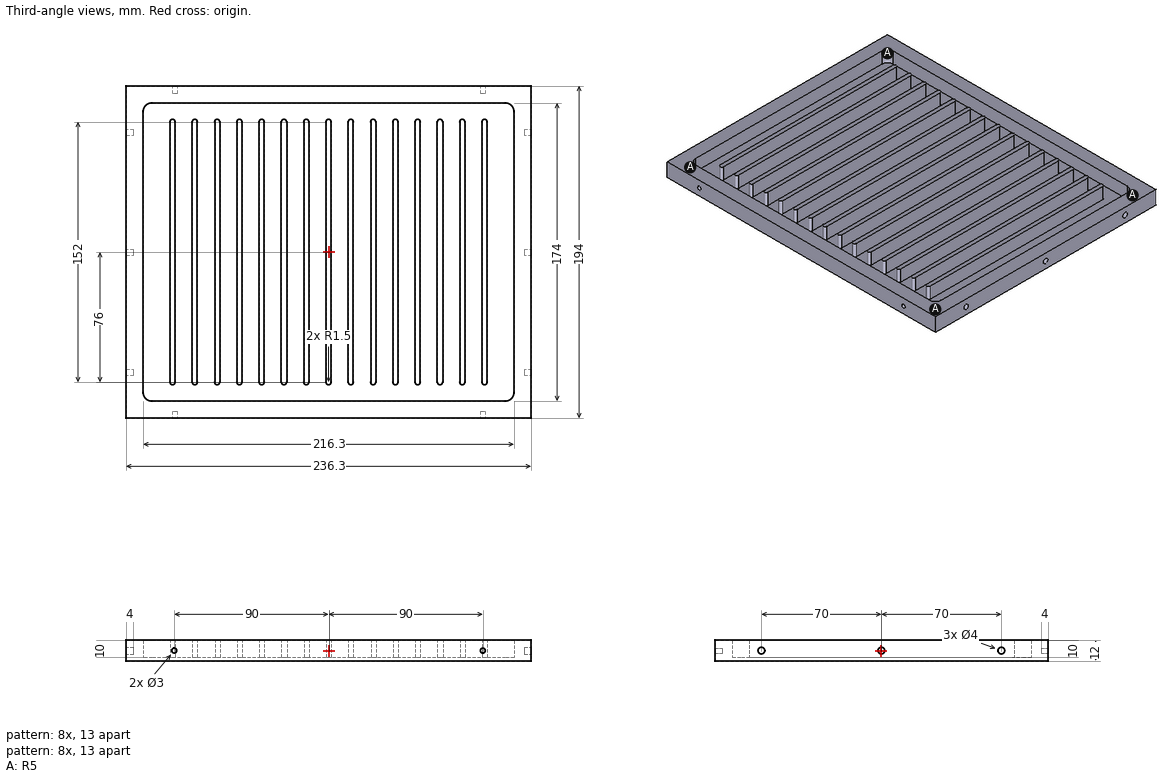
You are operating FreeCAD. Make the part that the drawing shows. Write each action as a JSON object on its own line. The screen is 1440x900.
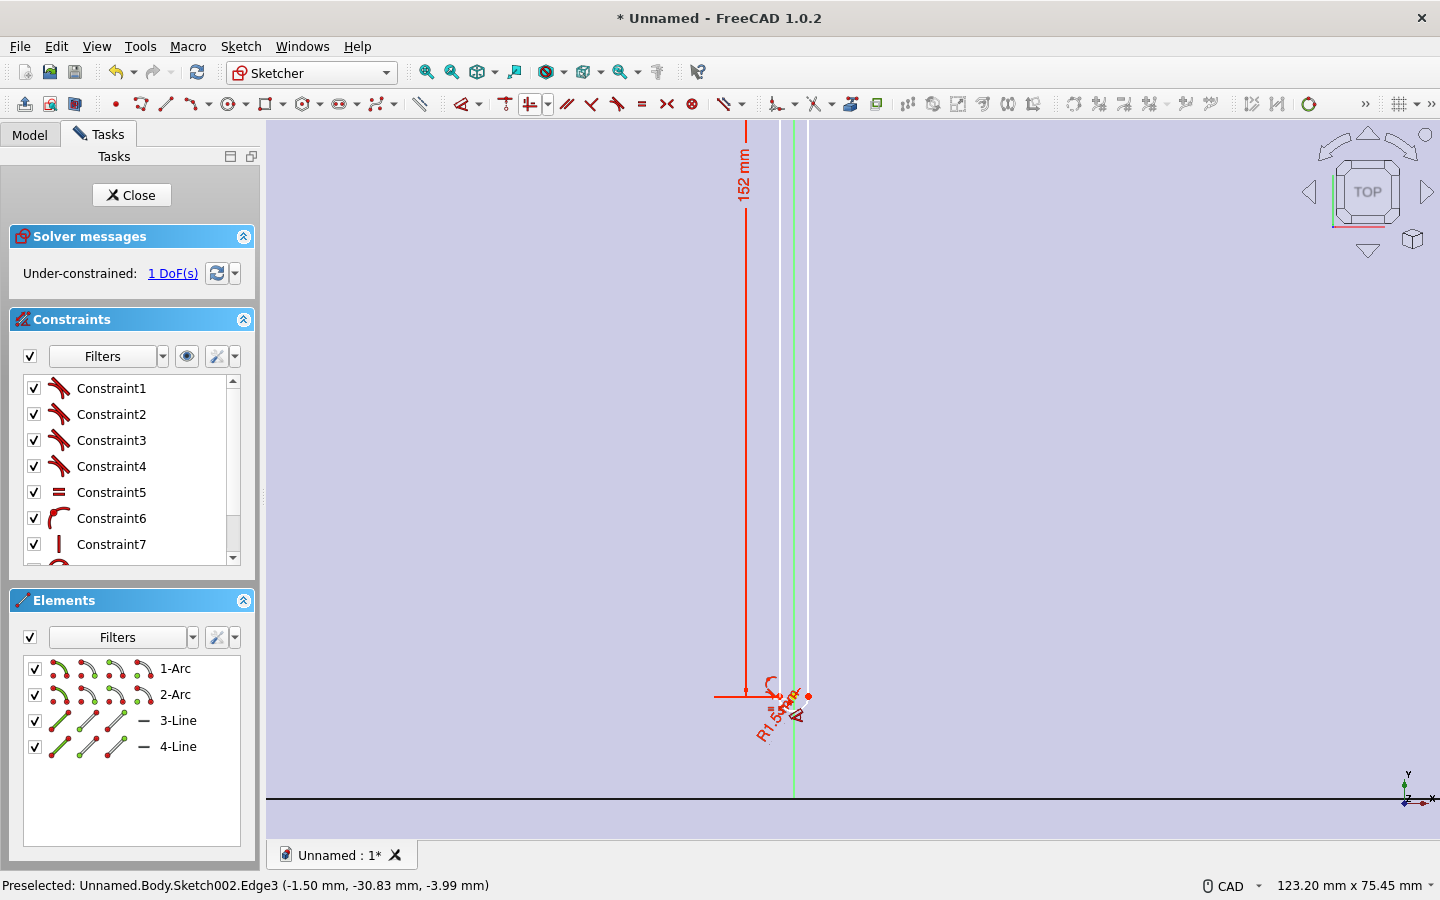
{"action": "left_click", "coordinate": [780, 697]}
{"action": "left_click", "coordinate": [746, 422]}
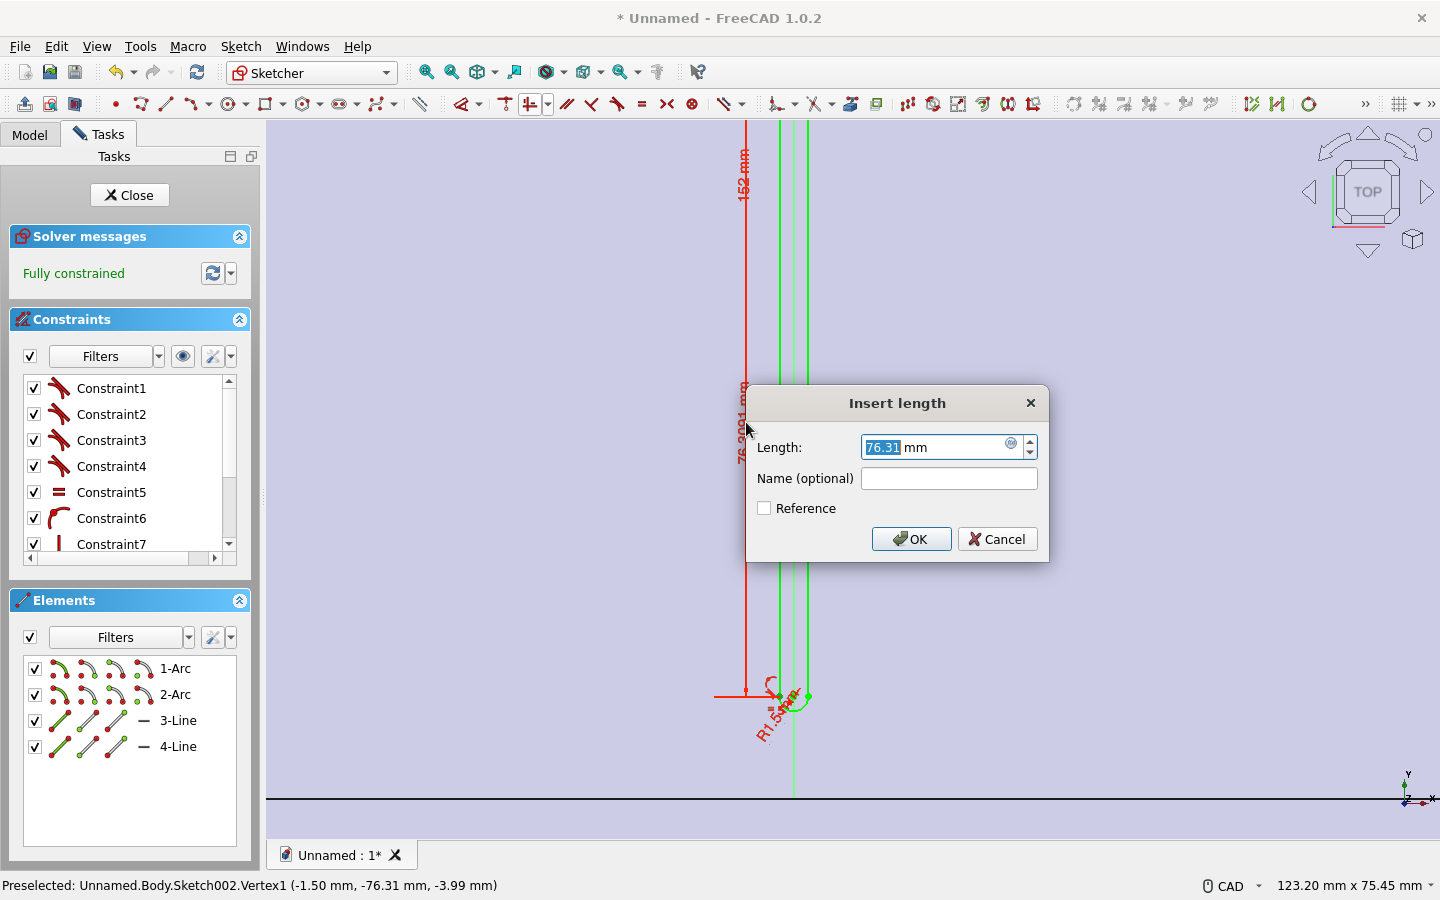
{"action": "type", "text": "76"}
{"action": "key", "text": "Return"}
{"action": "key", "text": "Escape"}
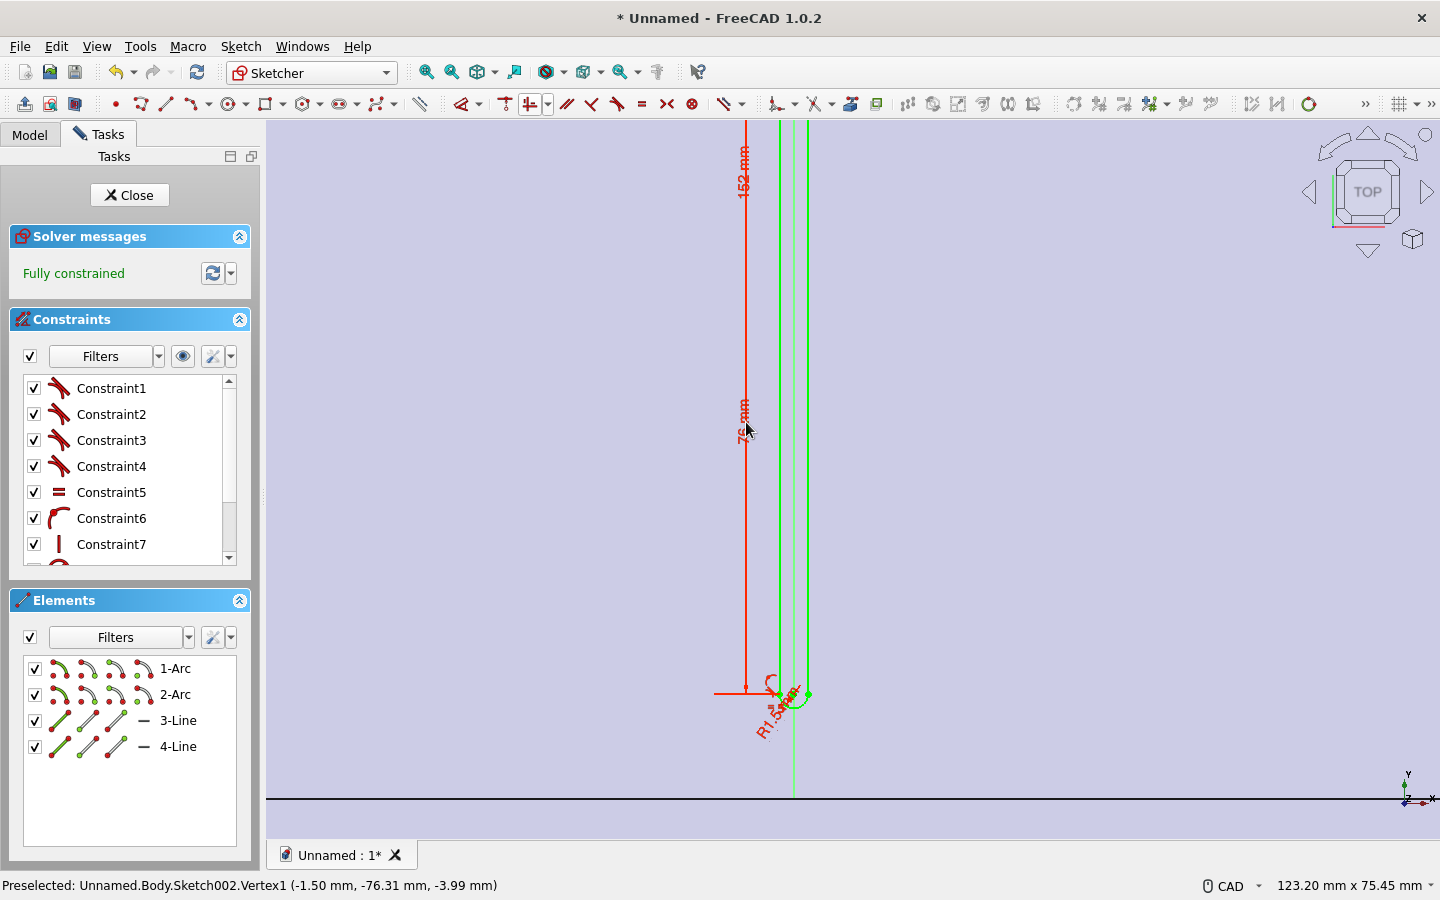
{"action": "left_click", "coordinate": [130, 195]}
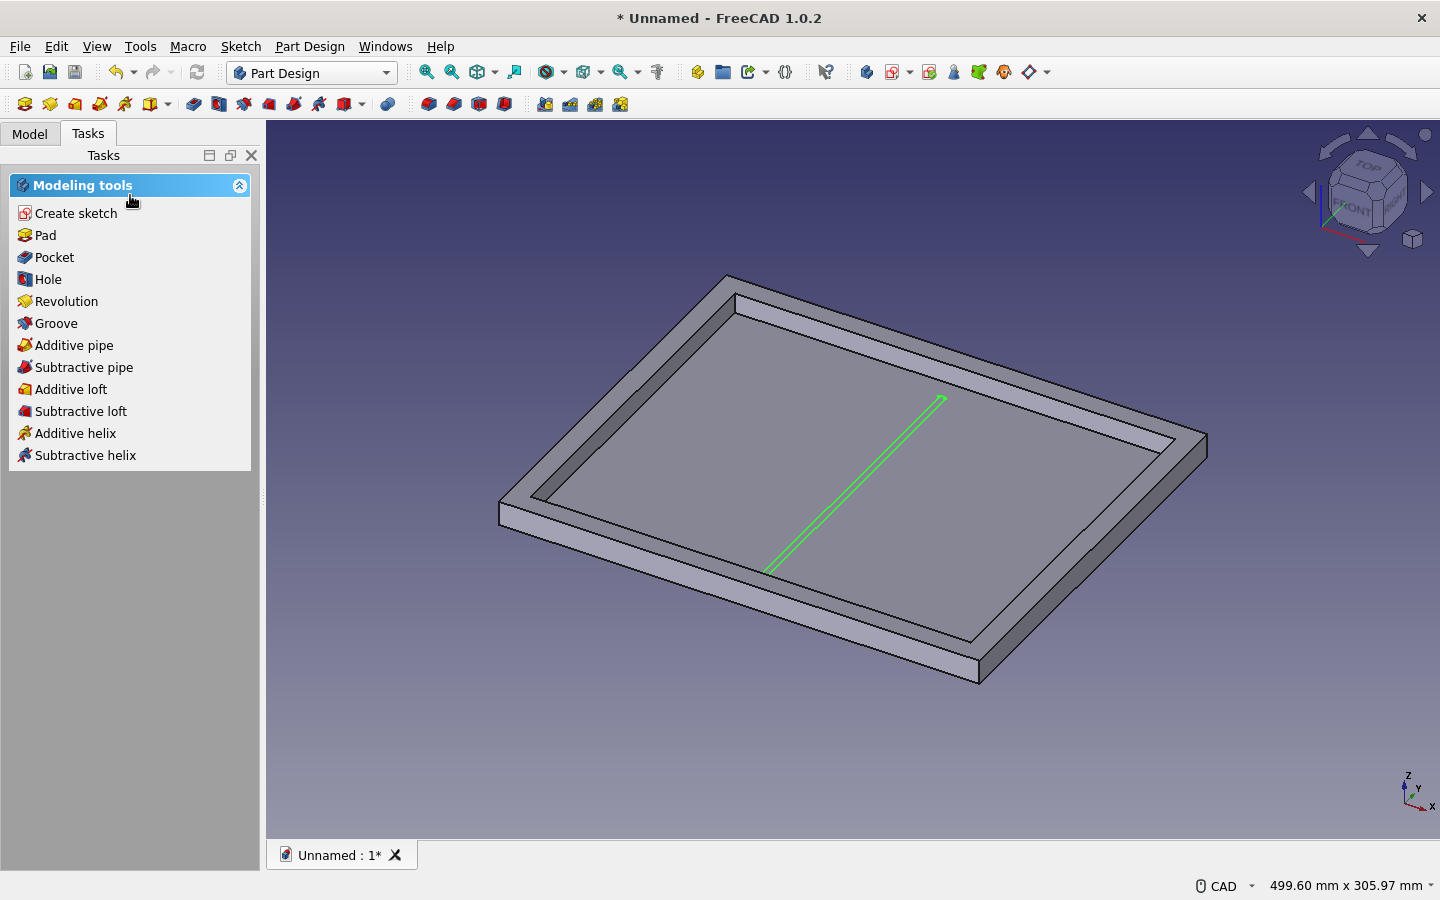
{"action": "left_click", "coordinate": [25, 104]}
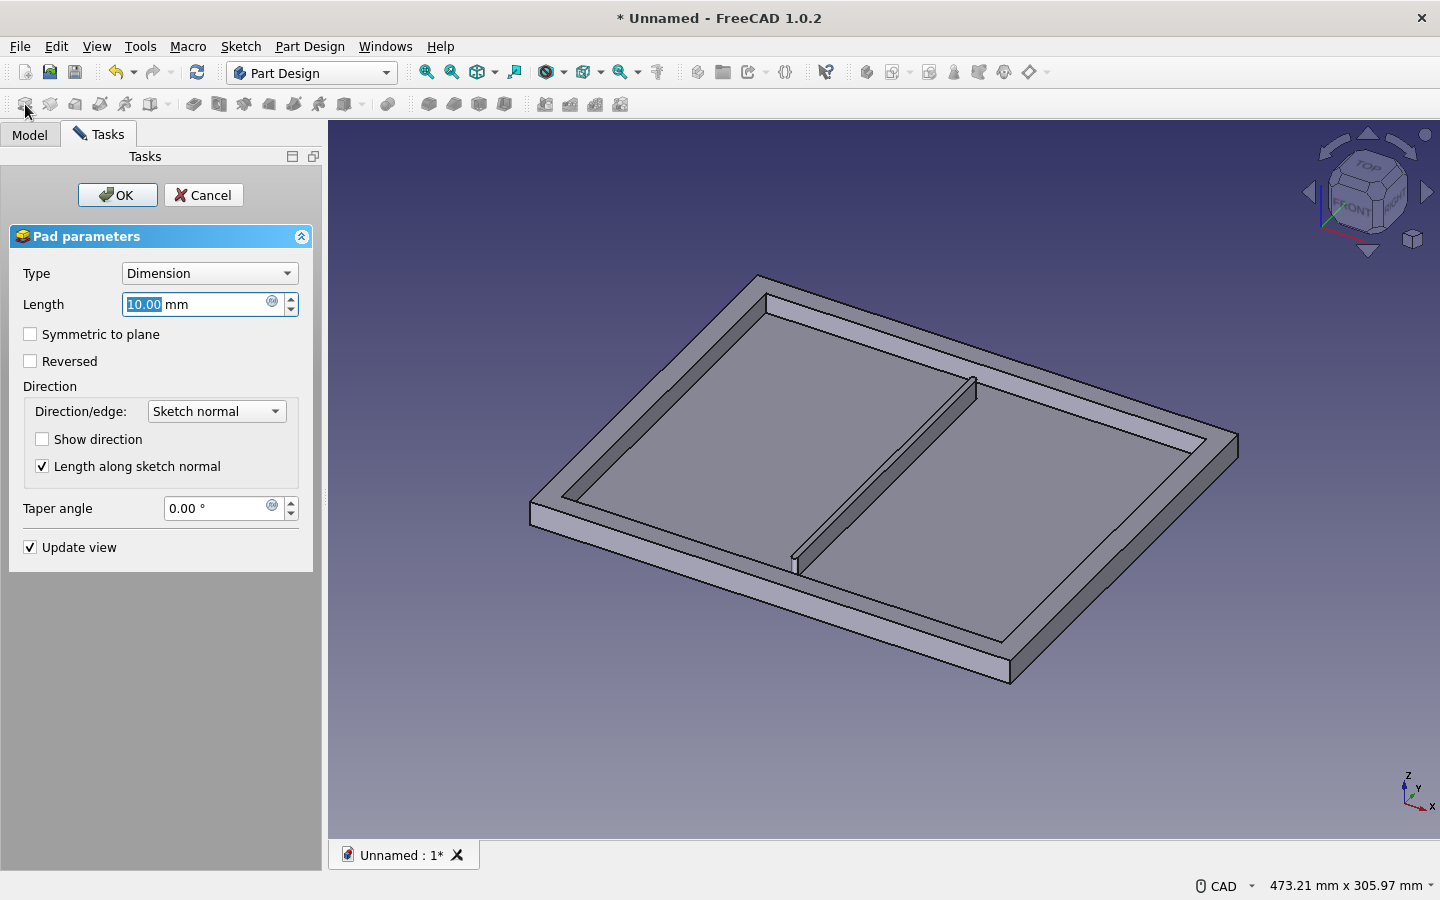
{"action": "type", "text": "10"}
{"action": "key", "text": "Tab"}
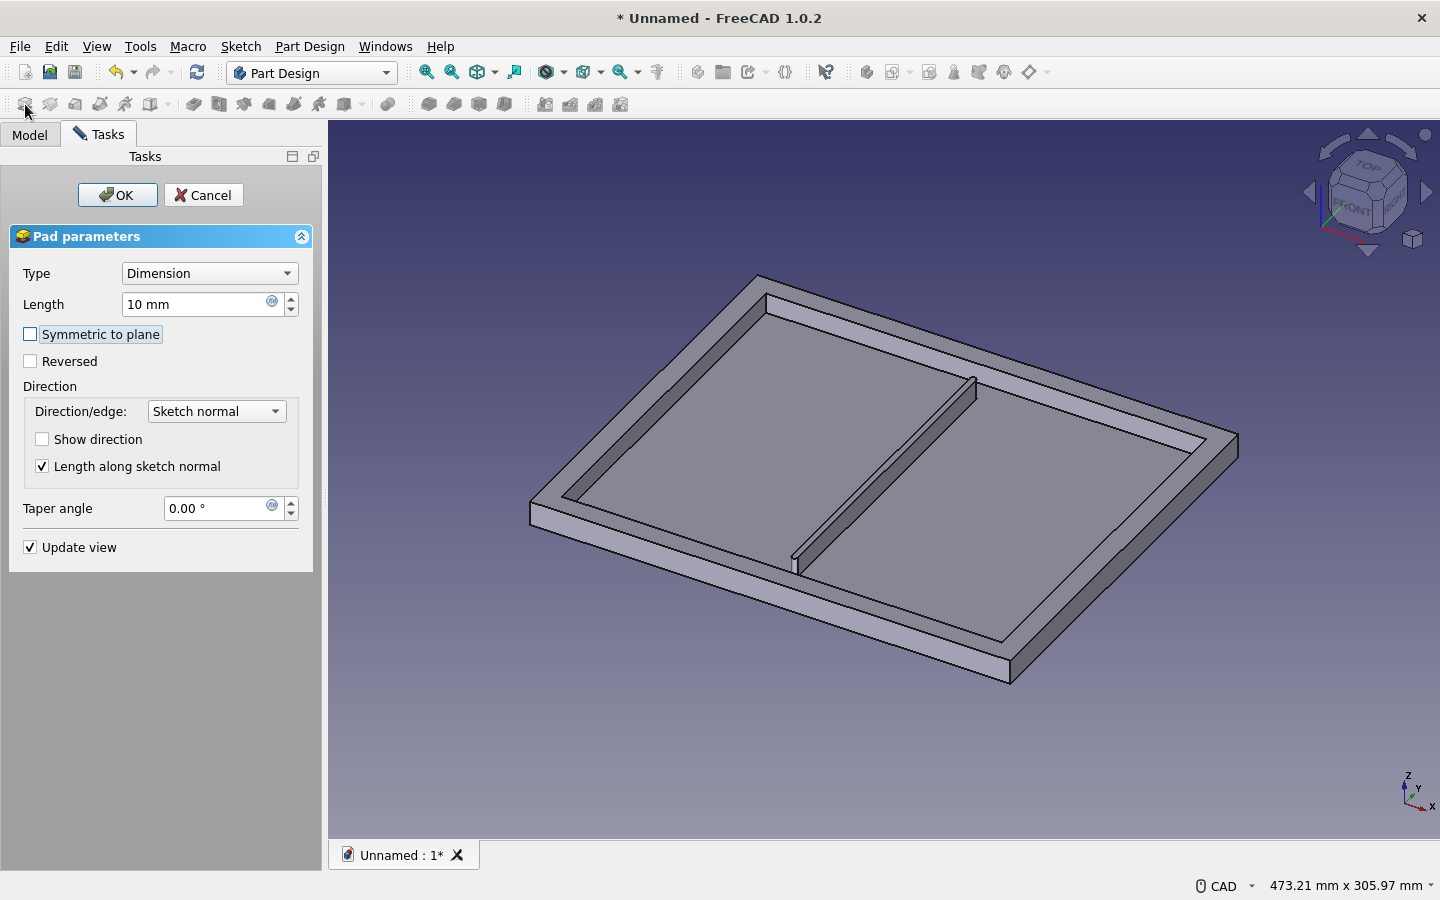
{"action": "left_click", "coordinate": [118, 195]}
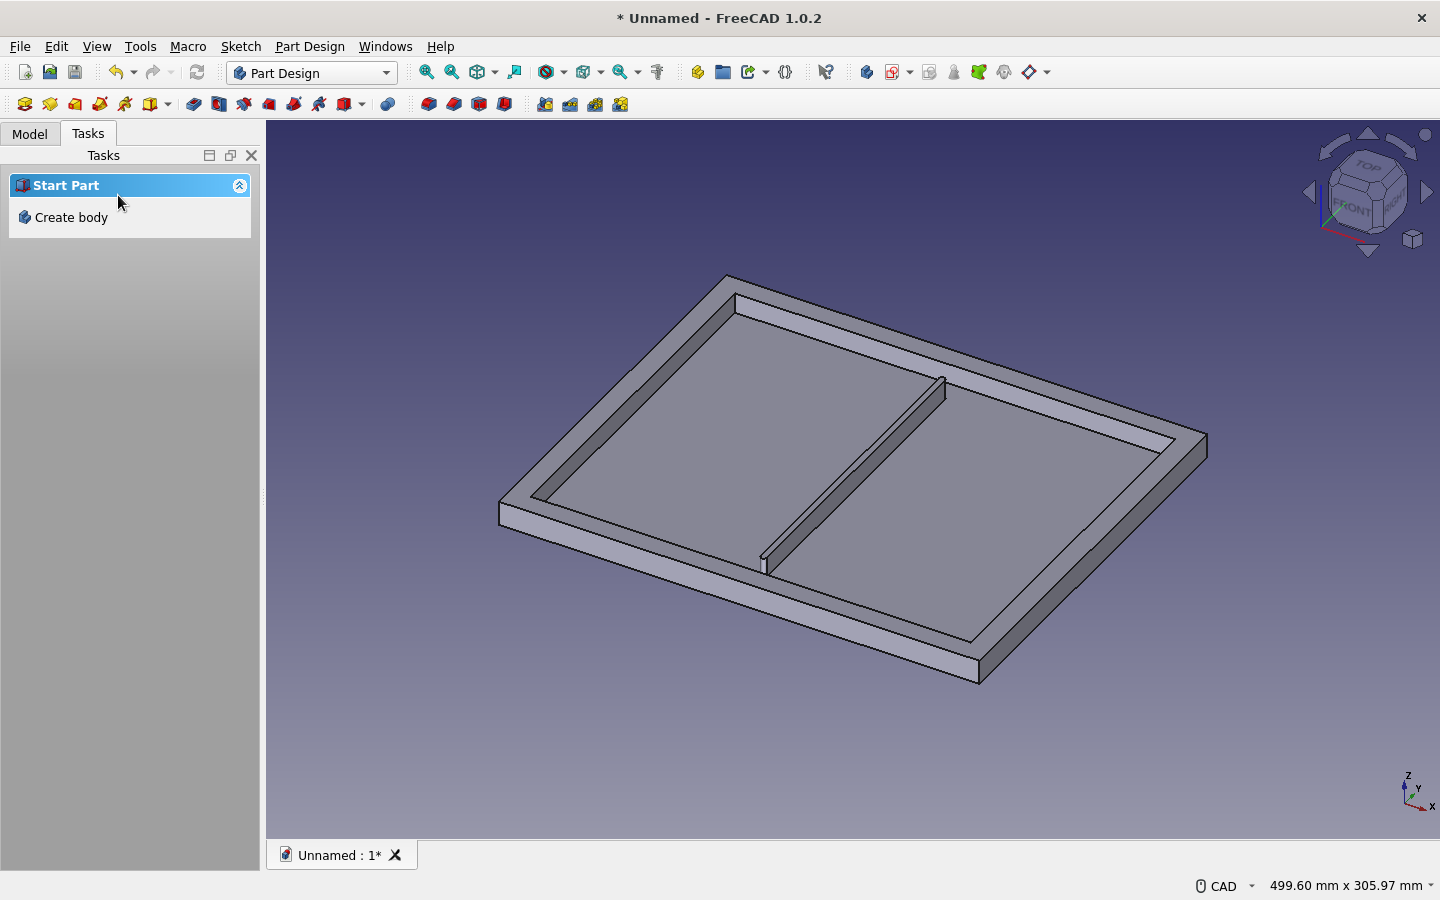
{"action": "left_click", "coordinate": [30, 134]}